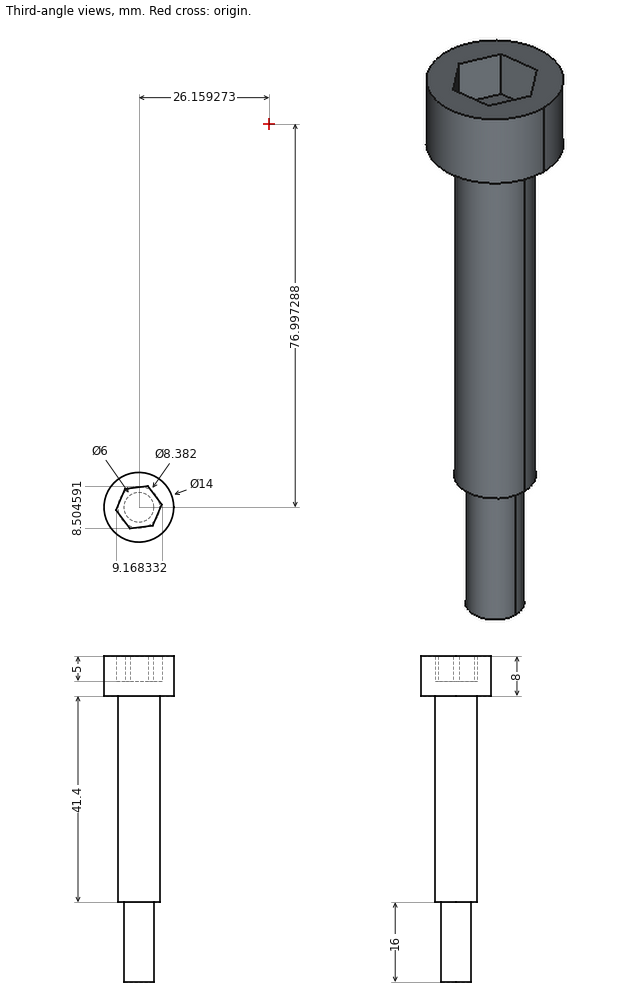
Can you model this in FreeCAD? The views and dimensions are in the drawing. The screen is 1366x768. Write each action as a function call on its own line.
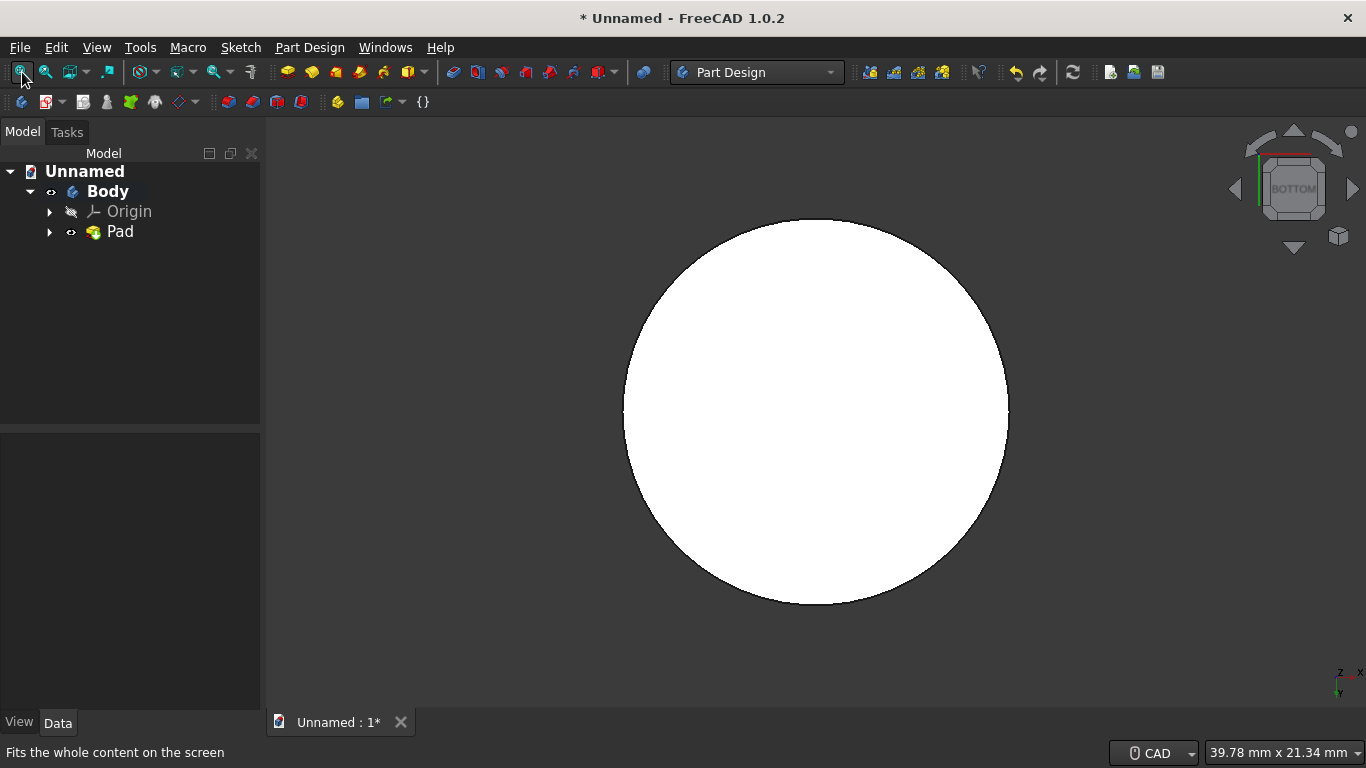
click(816, 411)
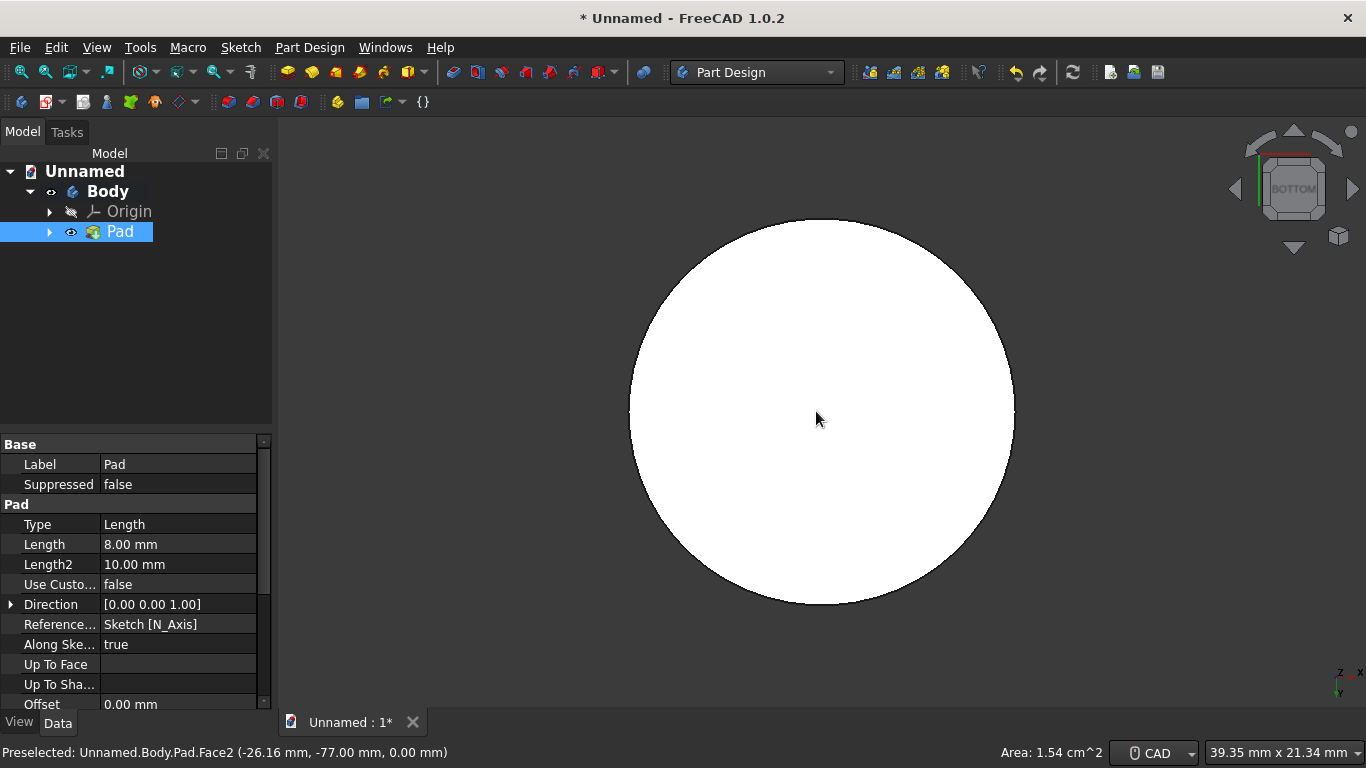
click(46, 102)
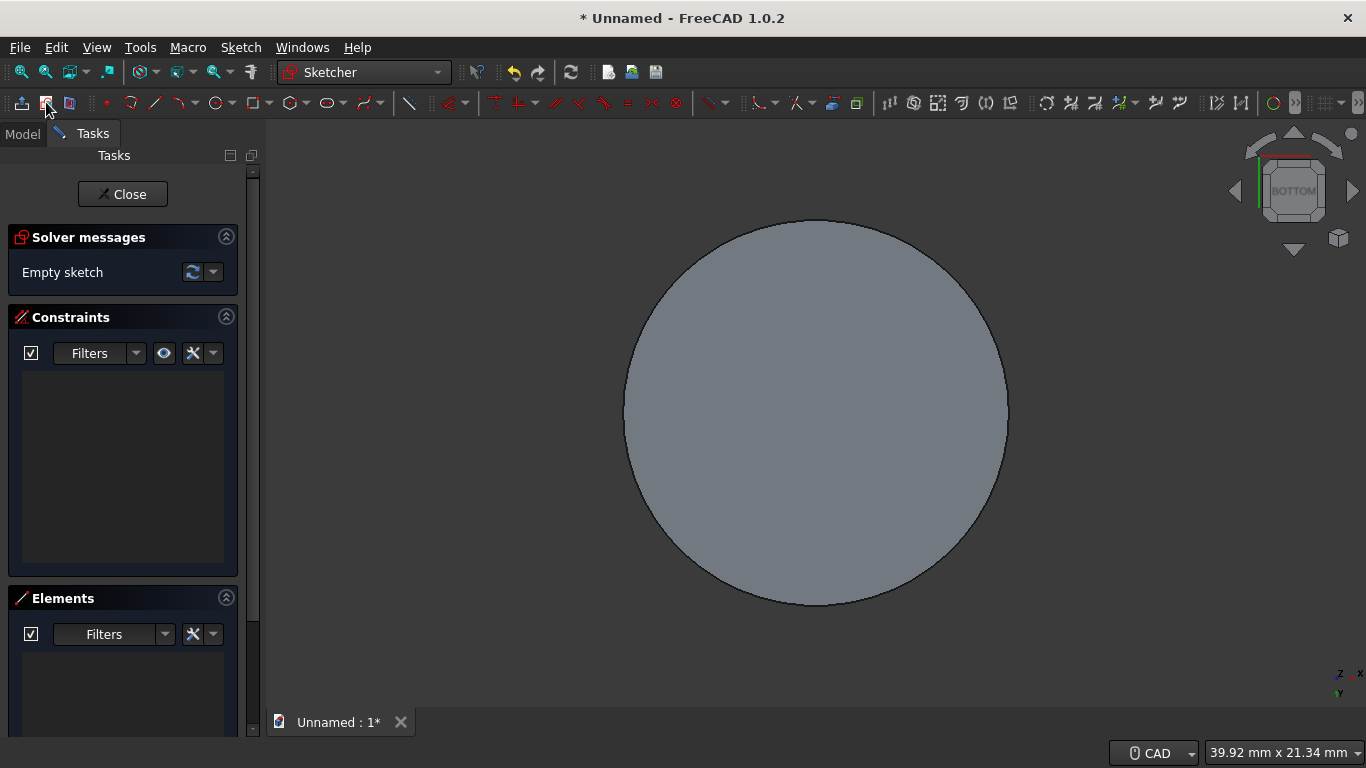
scroll(955, 413, up, 2)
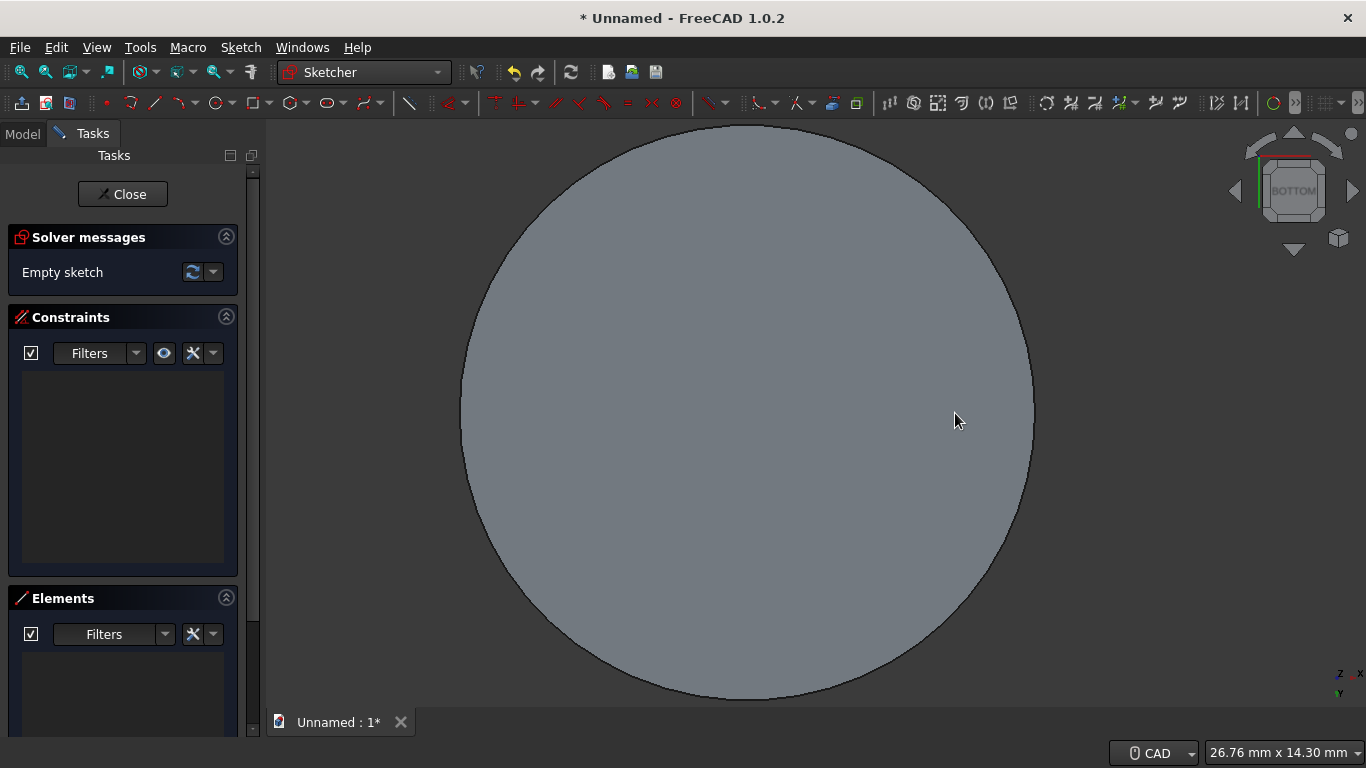
key(g)
key(c)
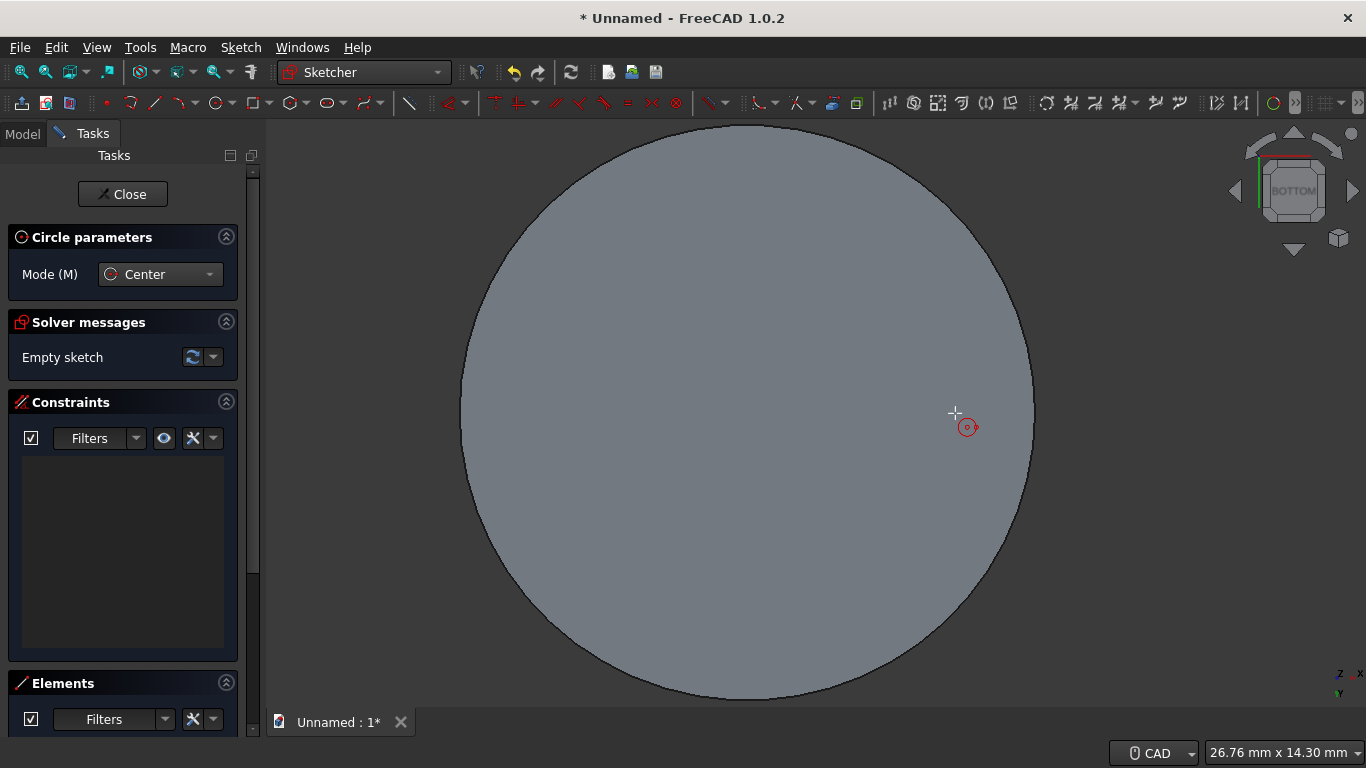
click(747, 413)
move(869, 291)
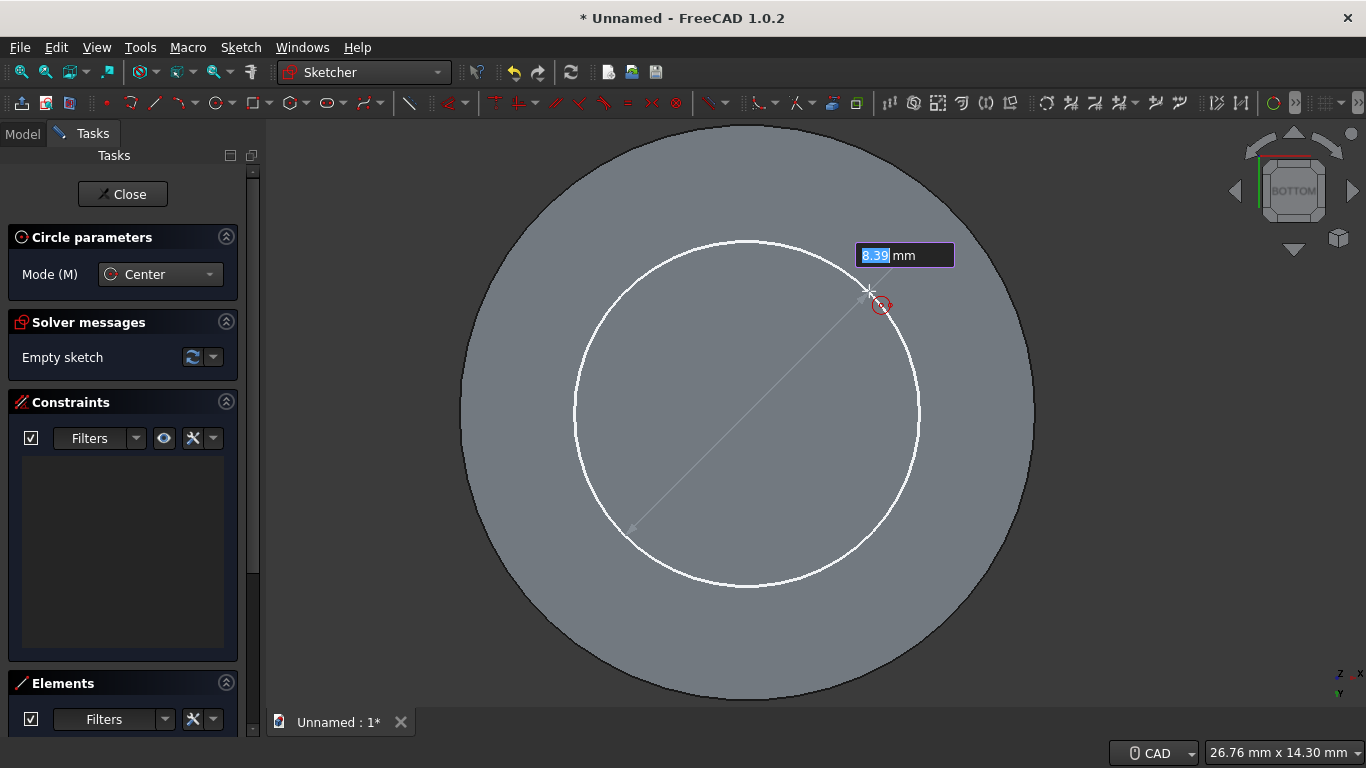
text(8.382)
key(Return)
key(Escape)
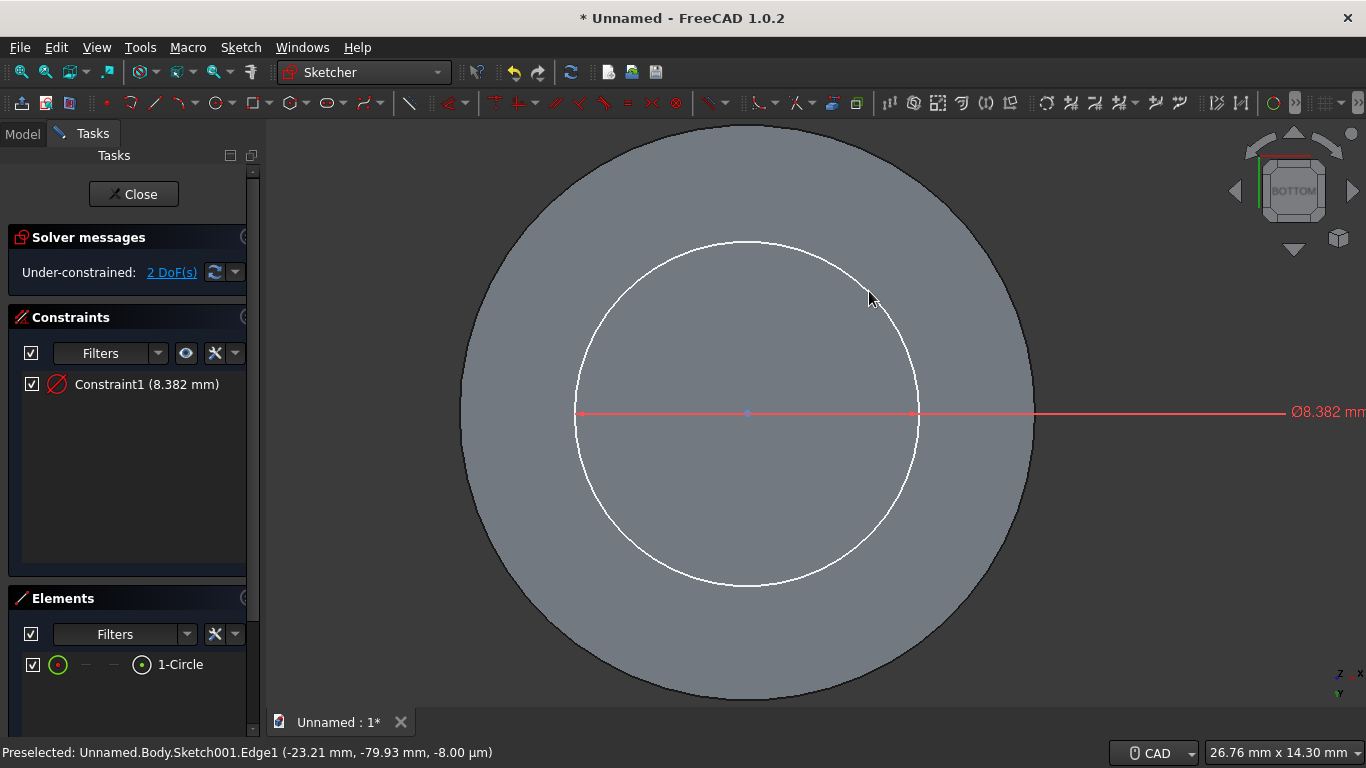
key(d)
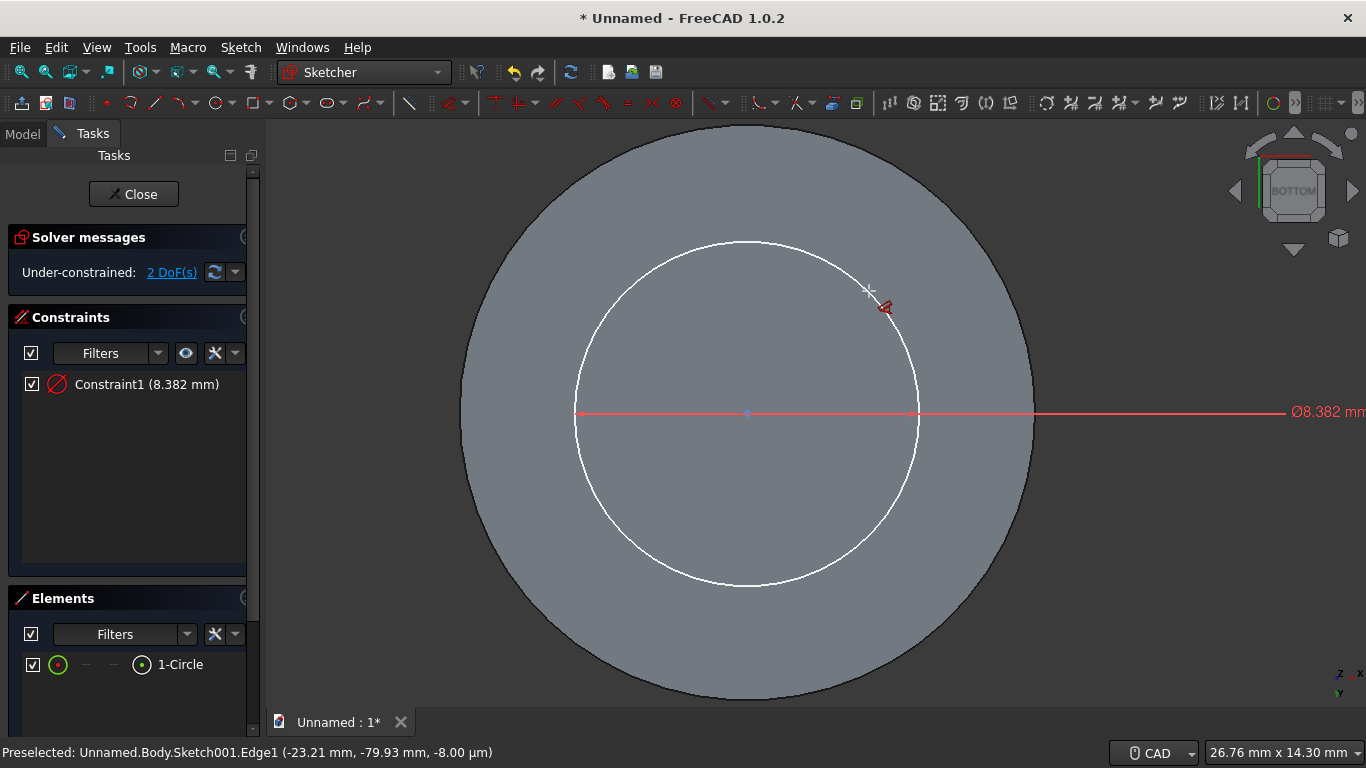
click(747, 414)
click(974, 380)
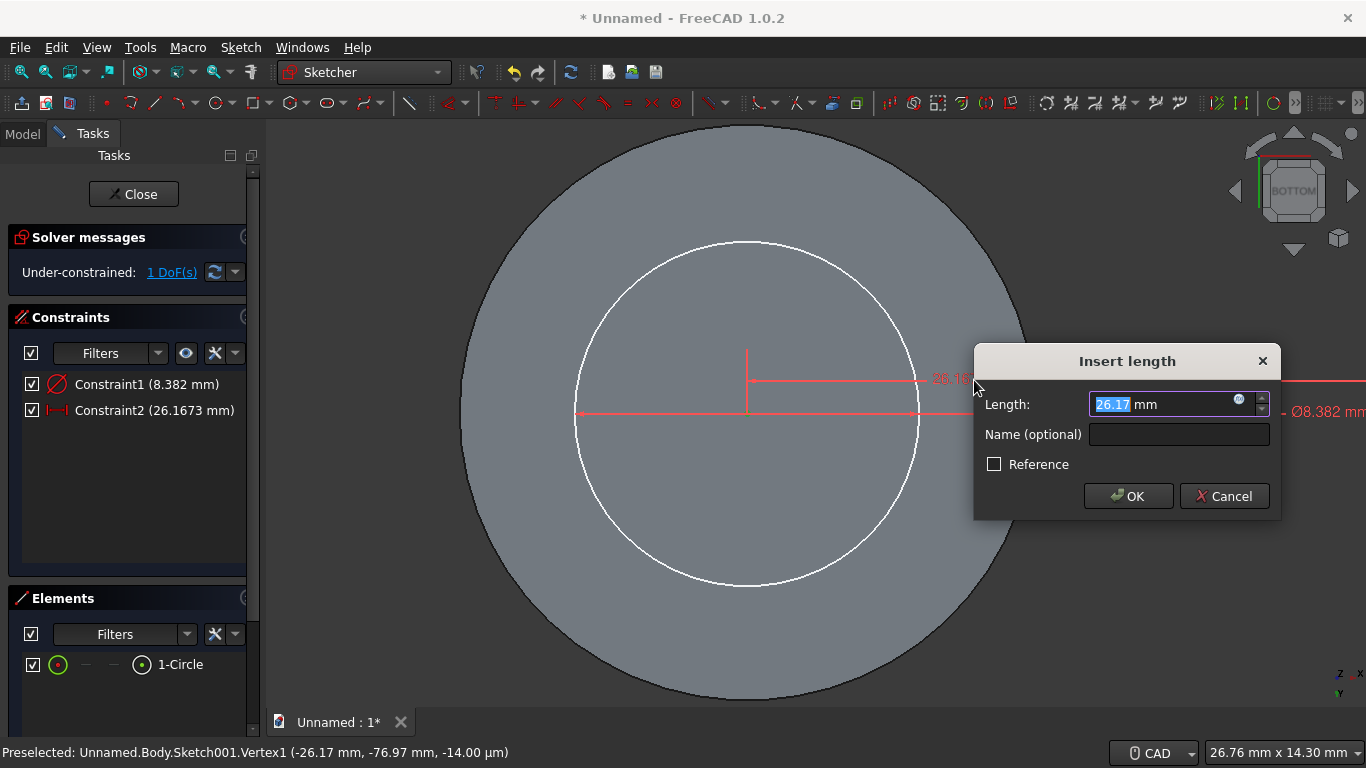
text(26.159273)
key(Return)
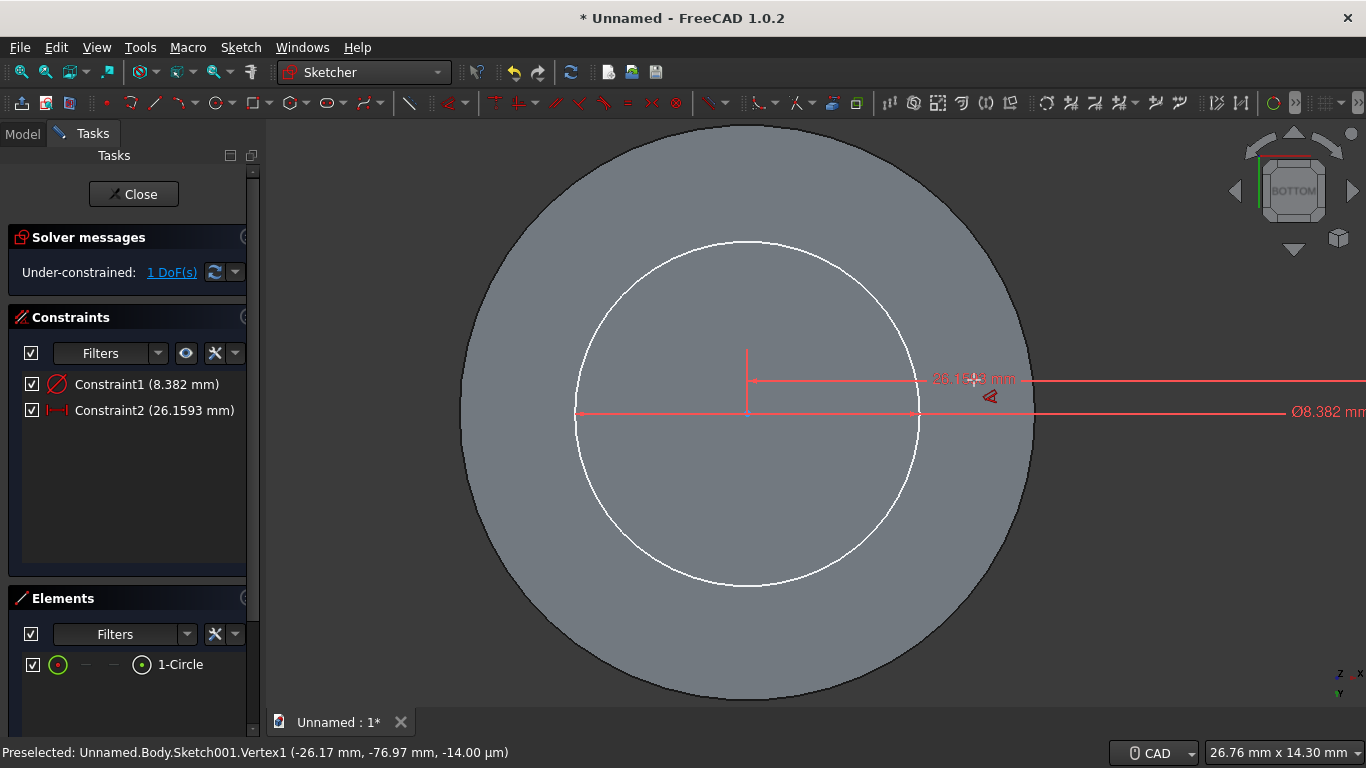
click(747, 414)
click(713, 546)